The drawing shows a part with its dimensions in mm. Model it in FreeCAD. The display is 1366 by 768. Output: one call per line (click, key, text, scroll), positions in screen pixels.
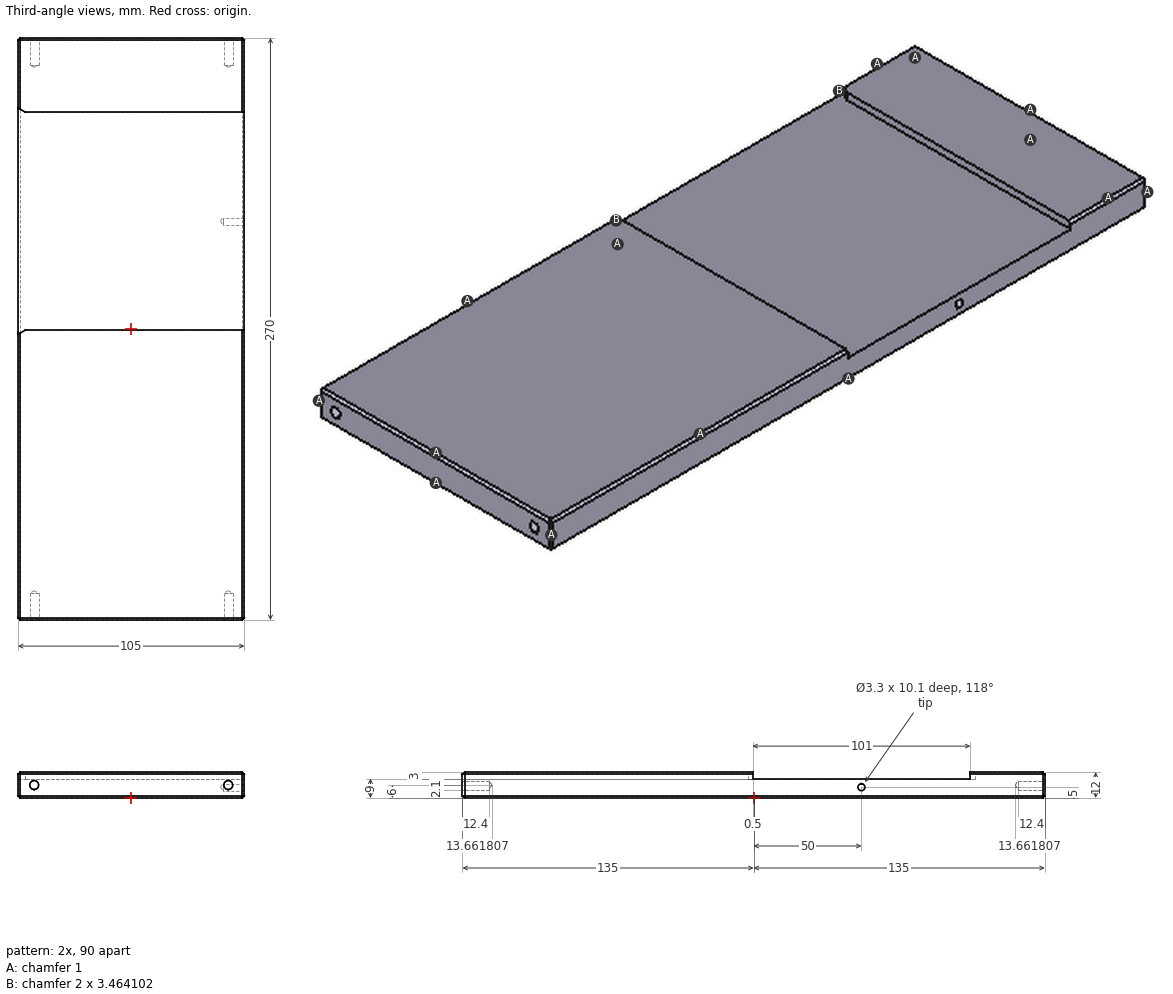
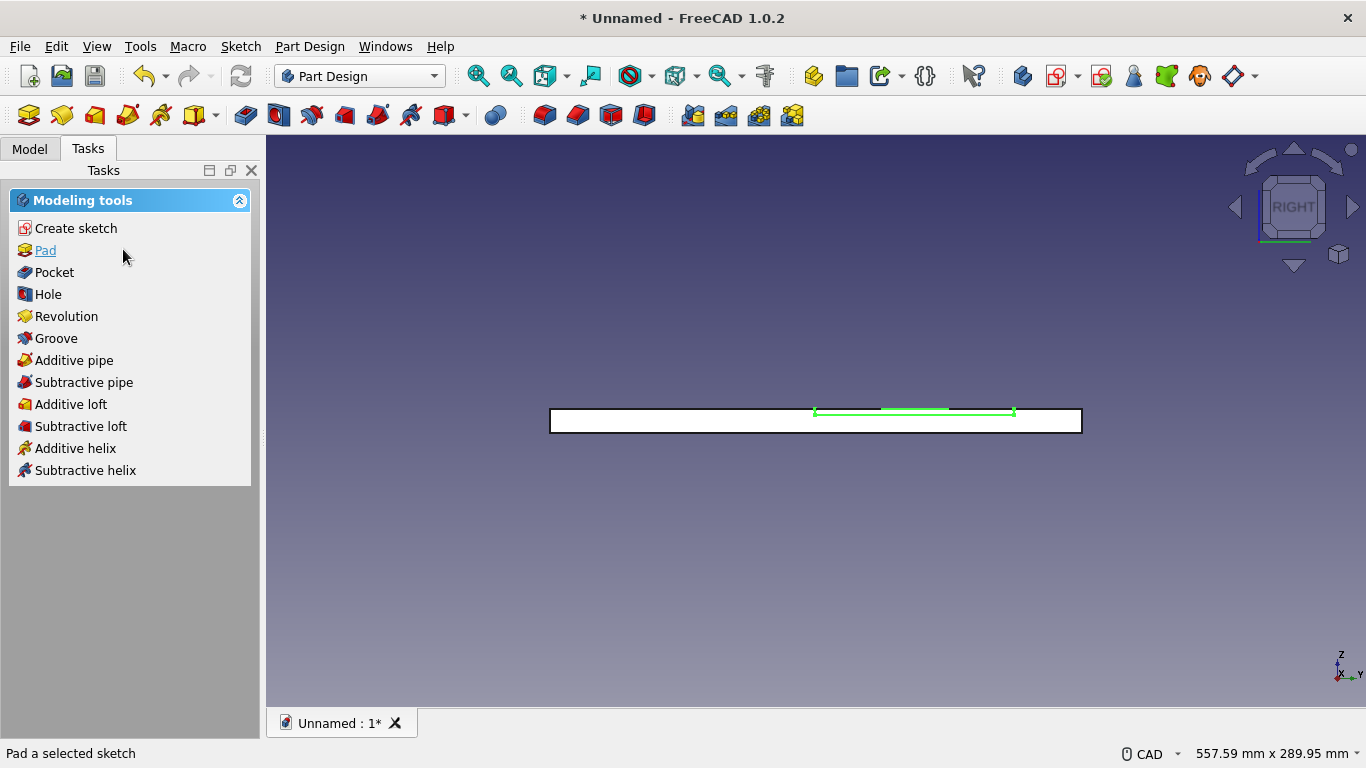
click(246, 116)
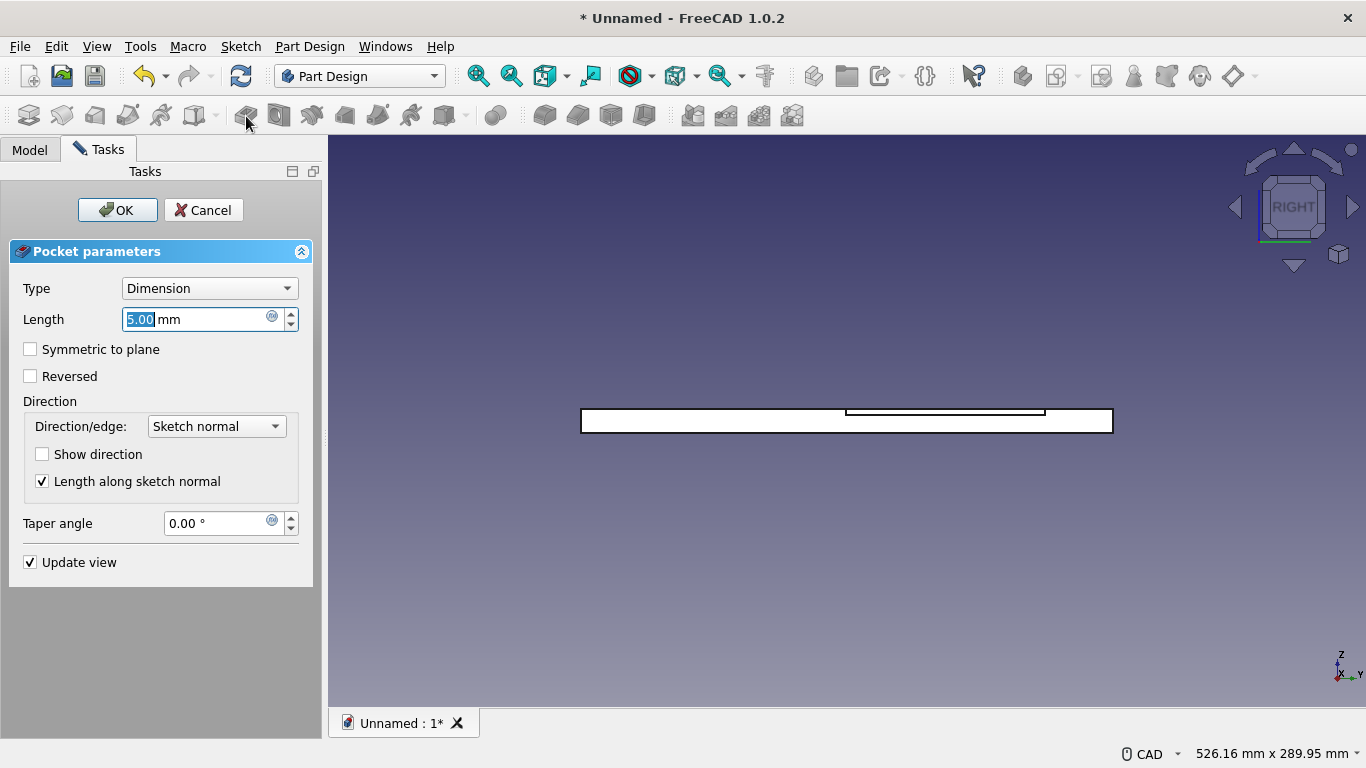
click(210, 288)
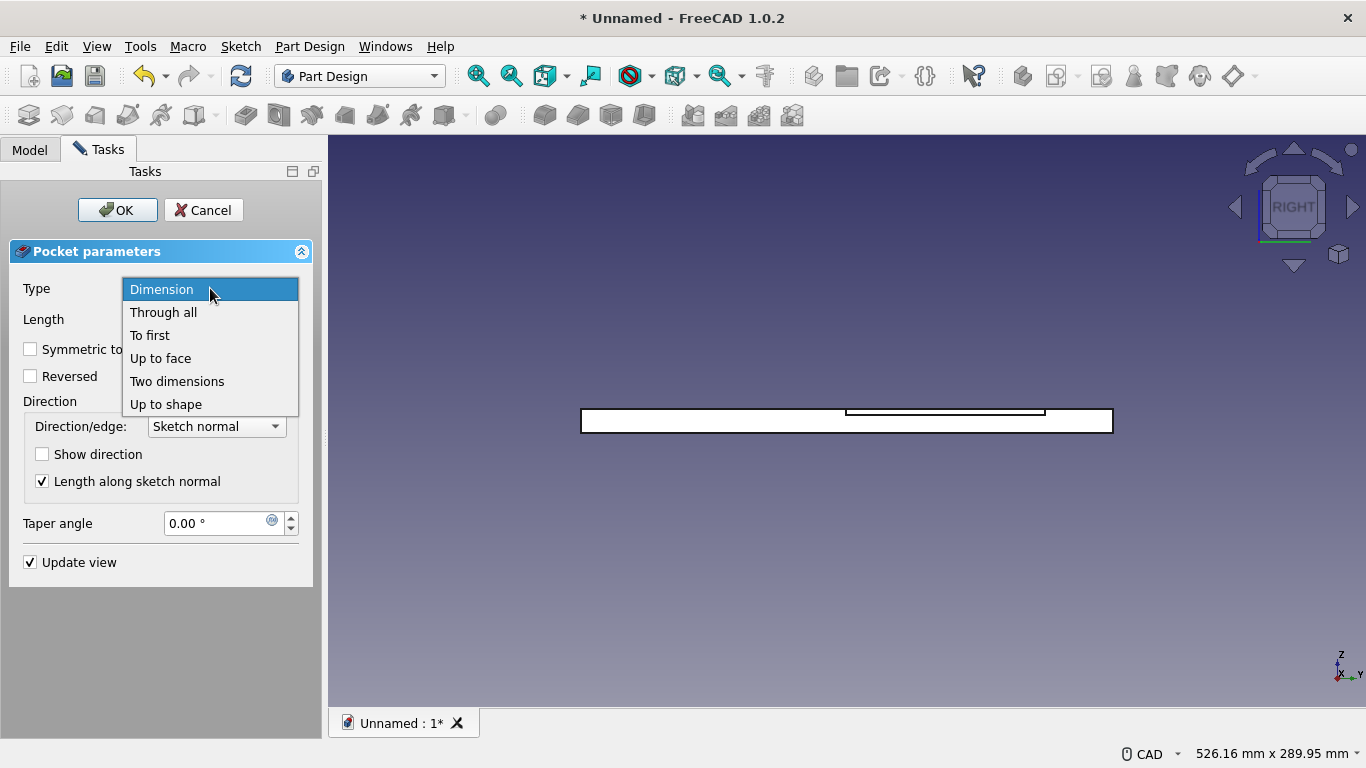
click(208, 312)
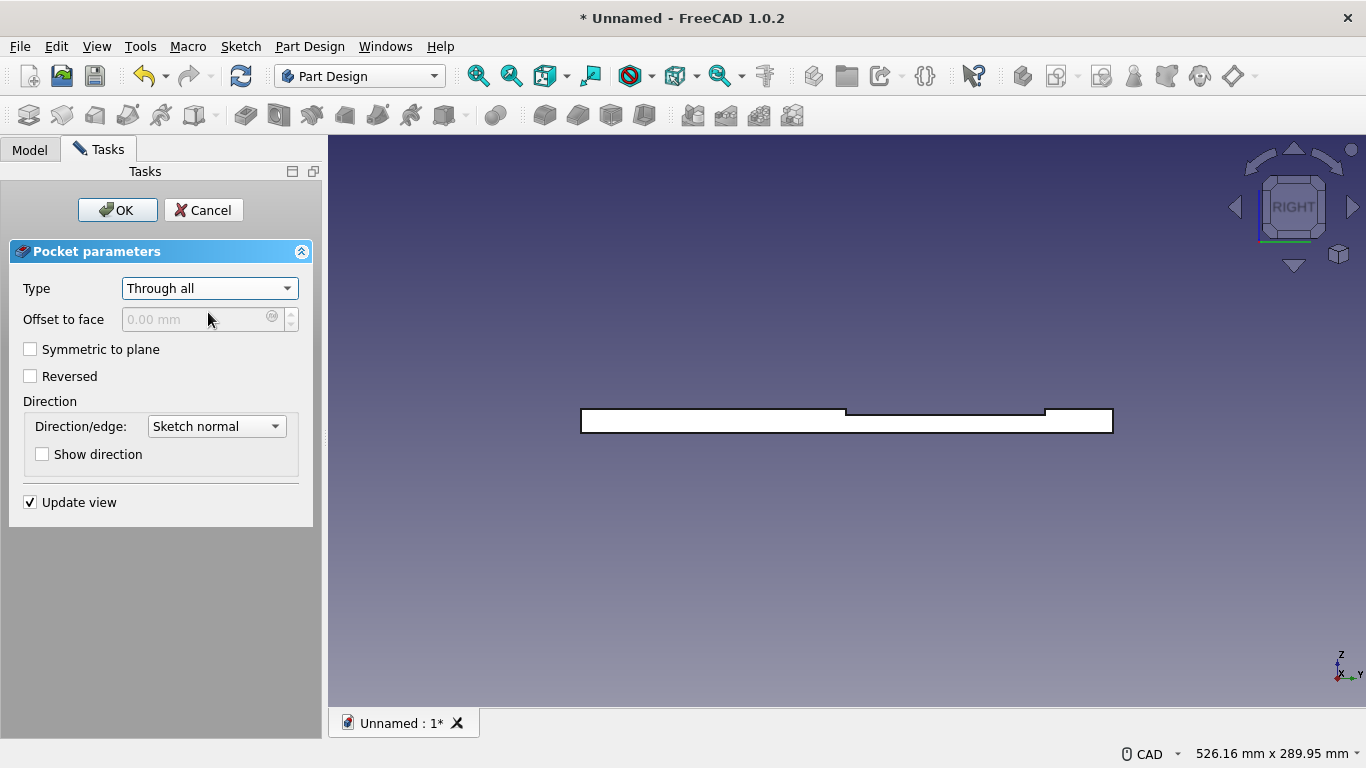
click(118, 210)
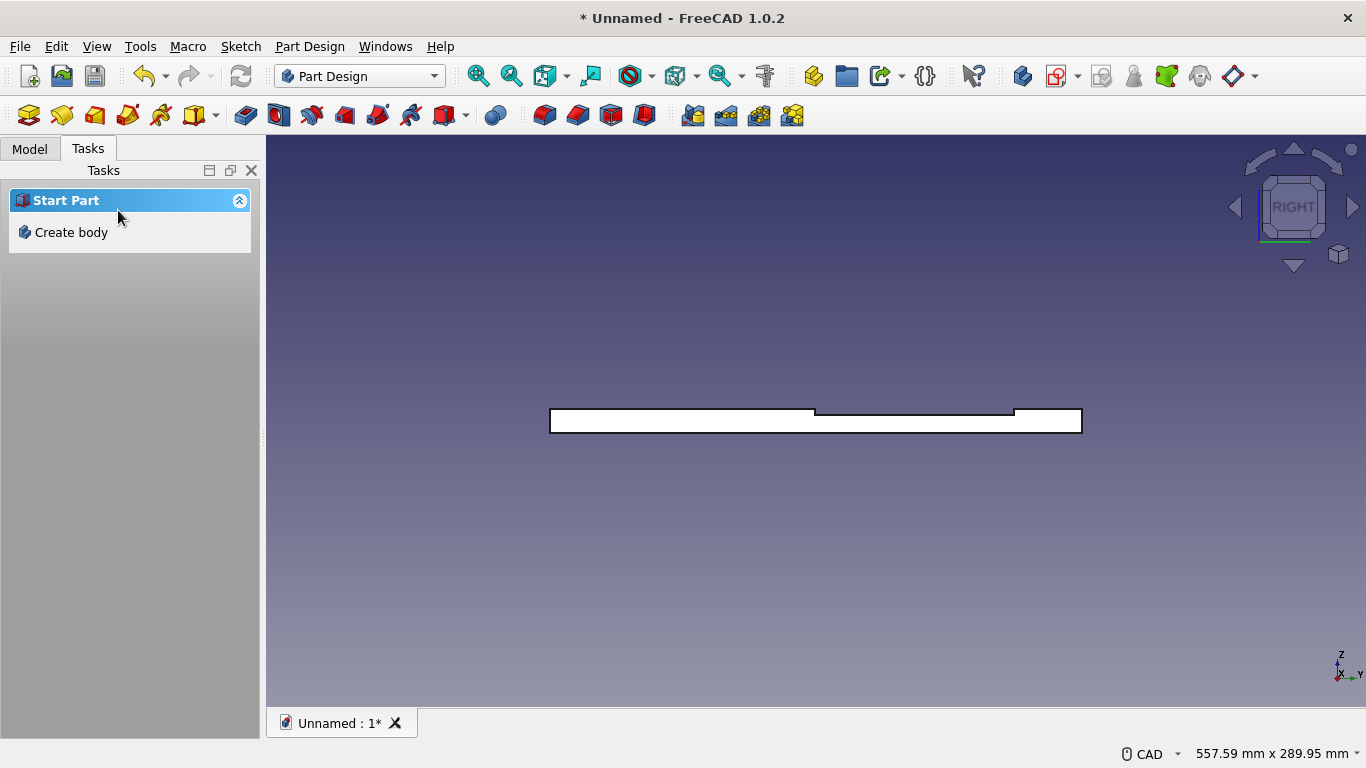
click(30, 148)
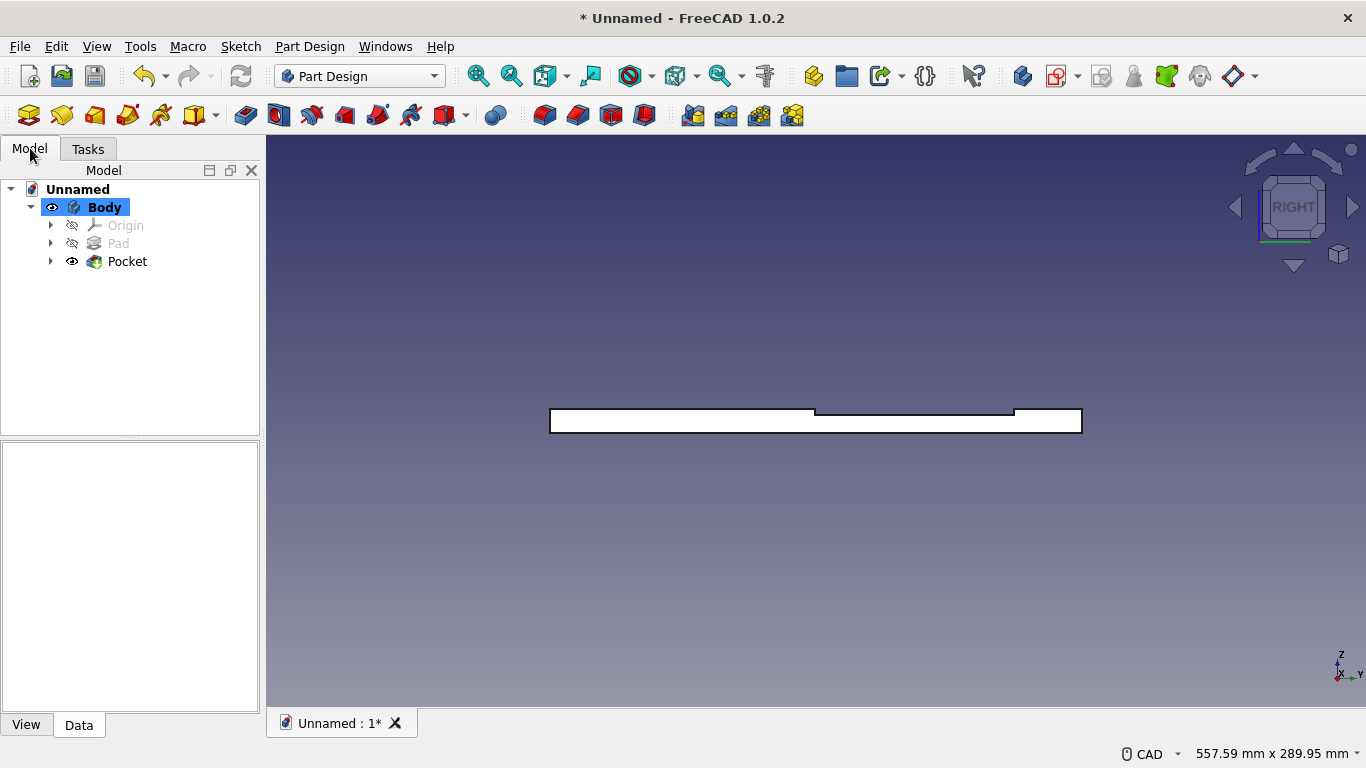
click(51, 225)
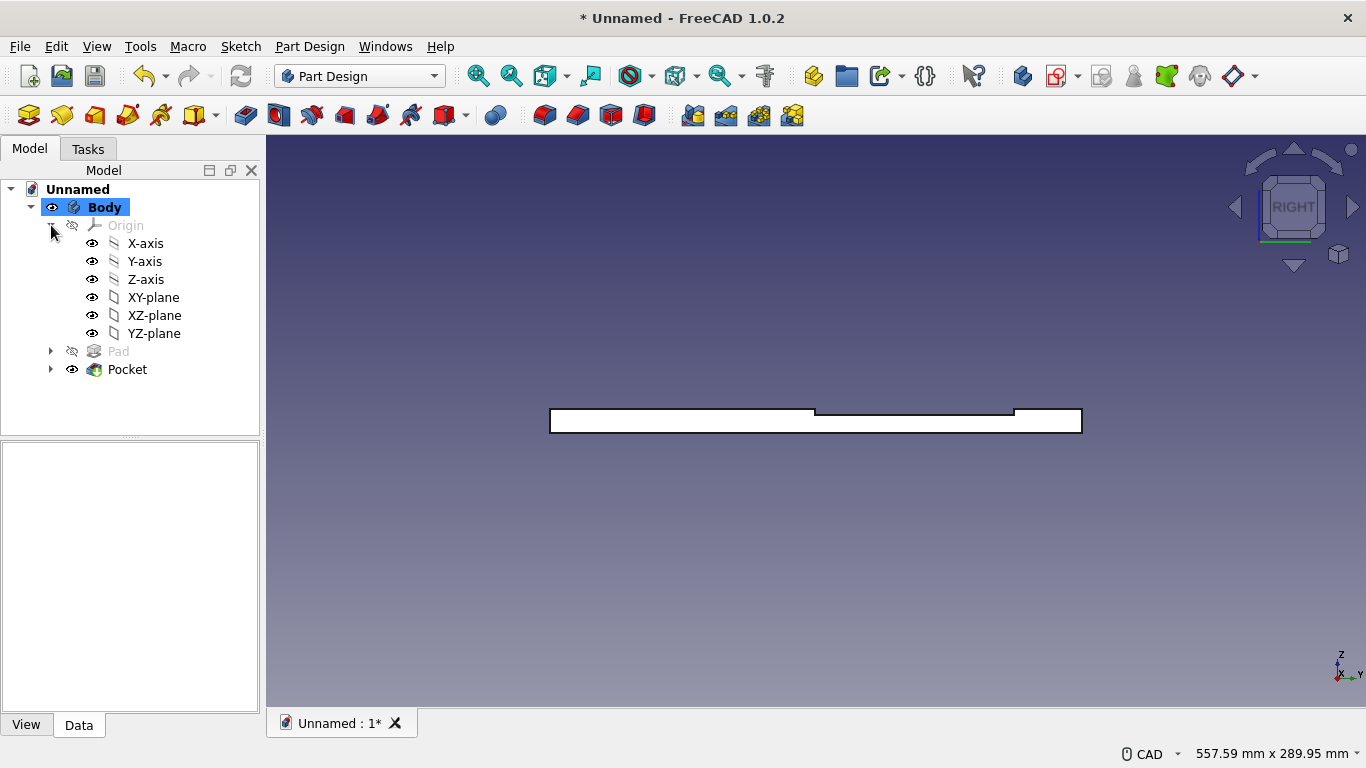
click(137, 333)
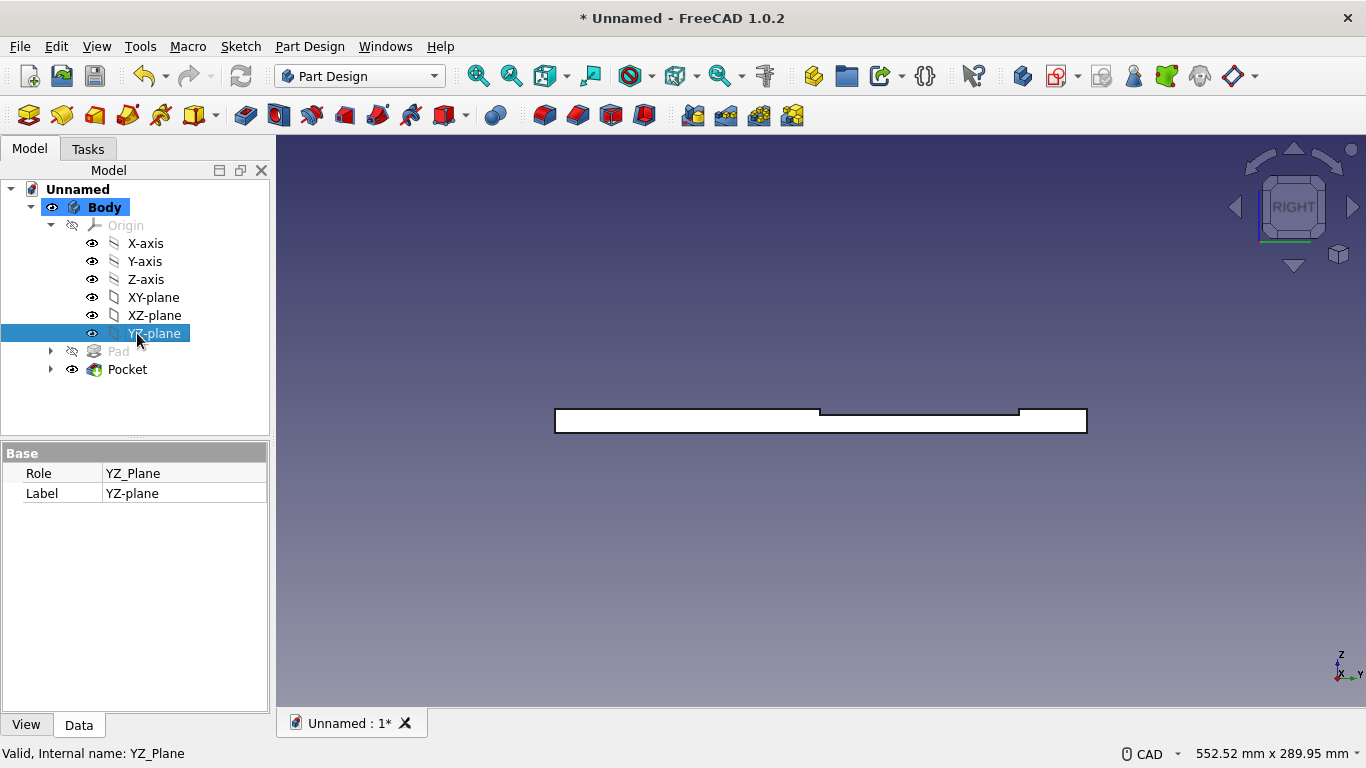
click(1232, 76)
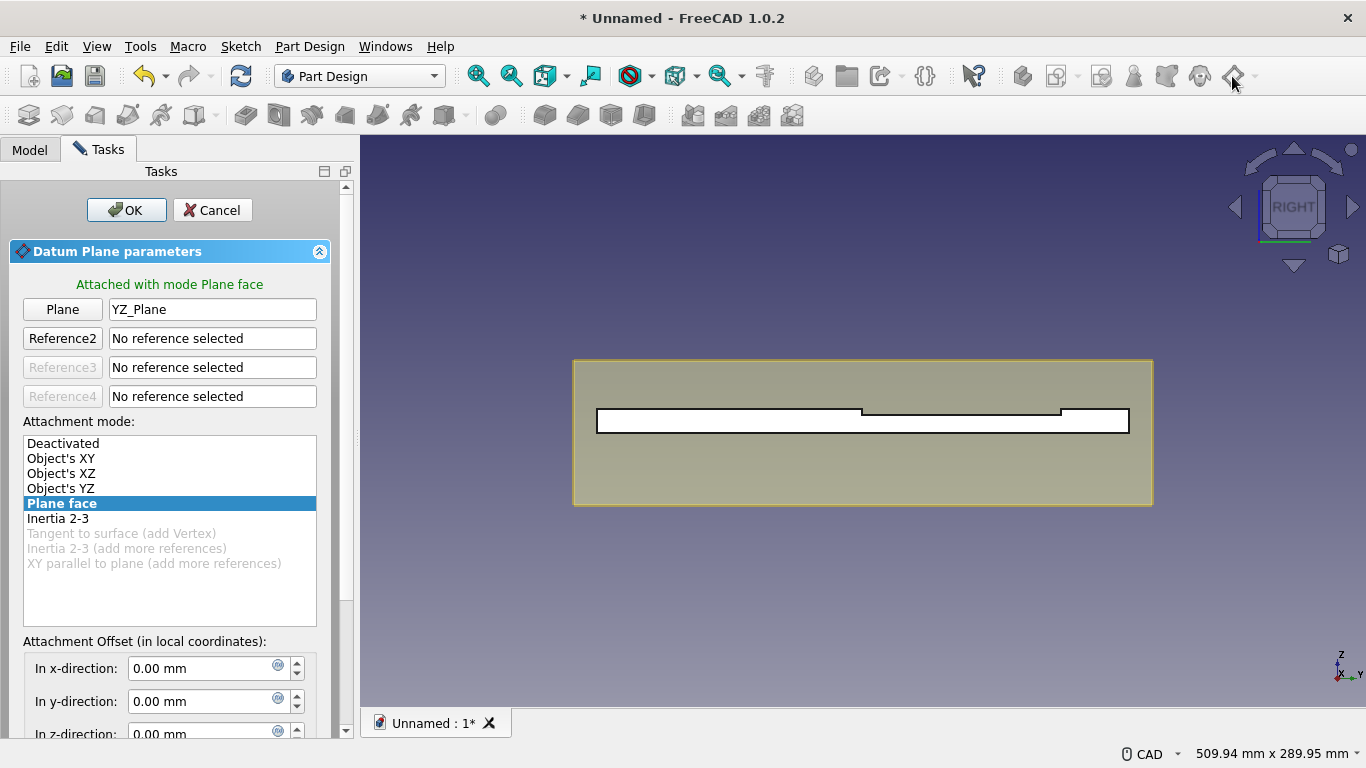
scroll(346, 460, down, 2)